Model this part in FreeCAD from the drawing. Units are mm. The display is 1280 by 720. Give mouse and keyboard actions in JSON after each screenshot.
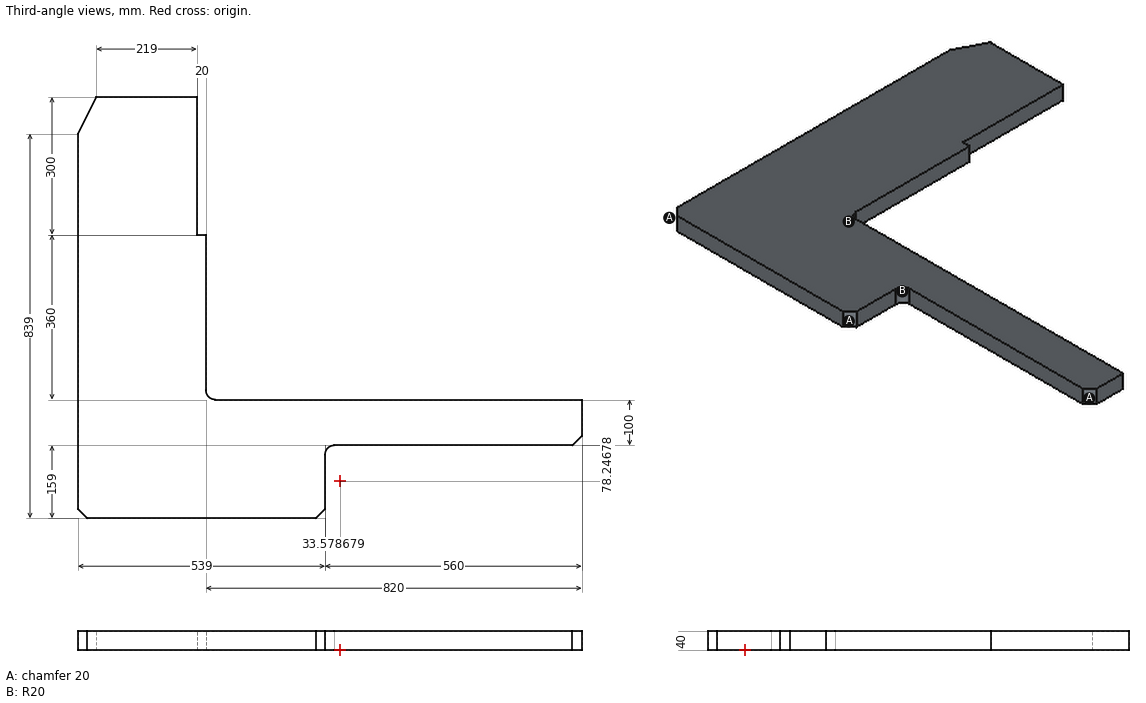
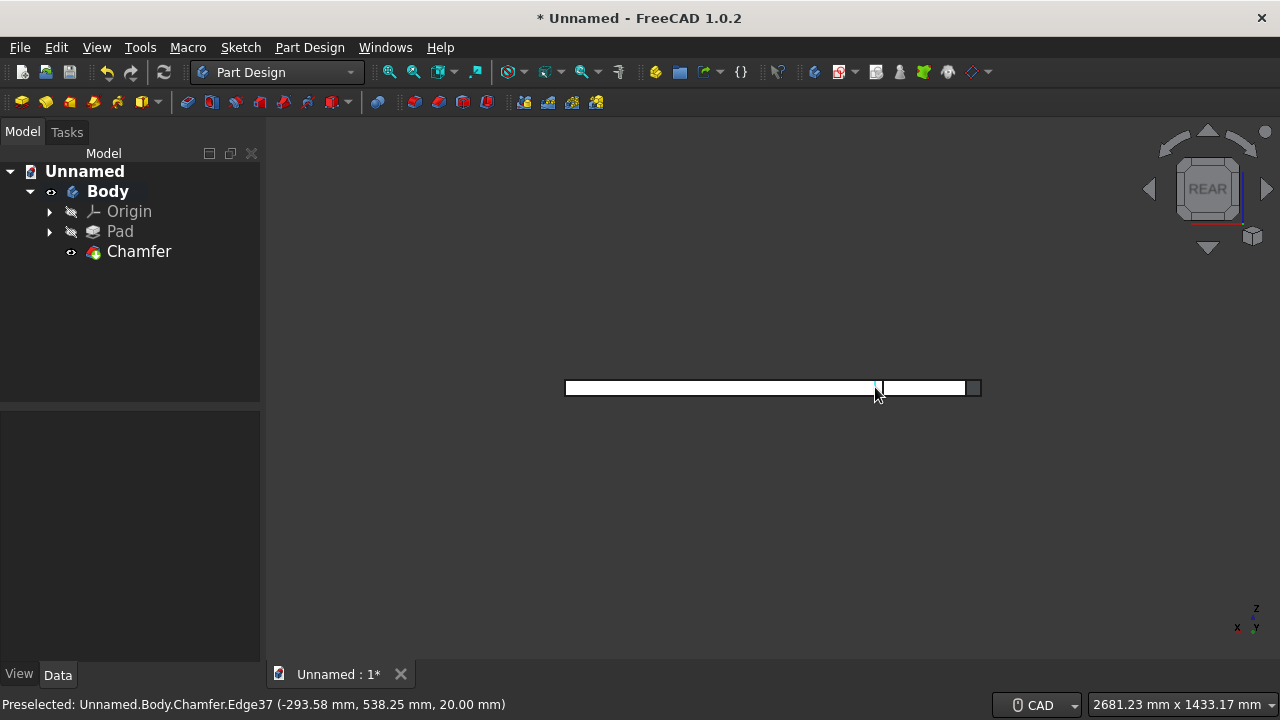
{"action": "key", "text": "6"}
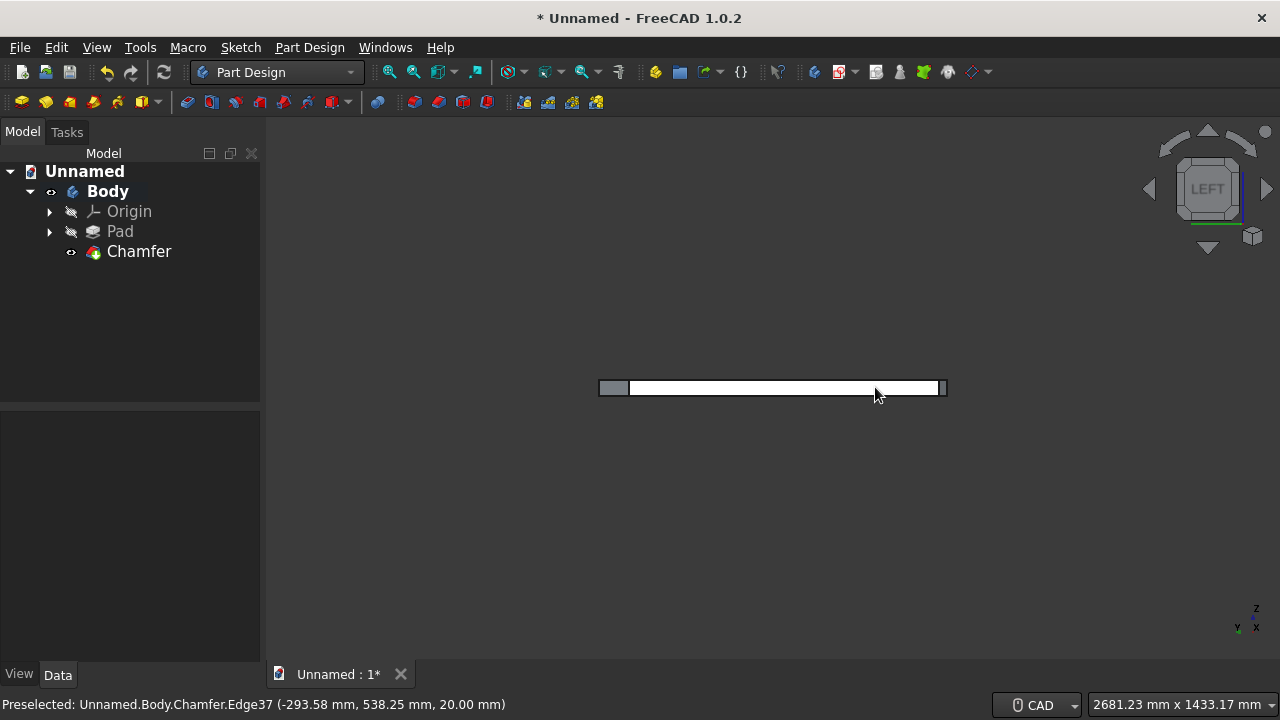
{"action": "key", "text": "v f"}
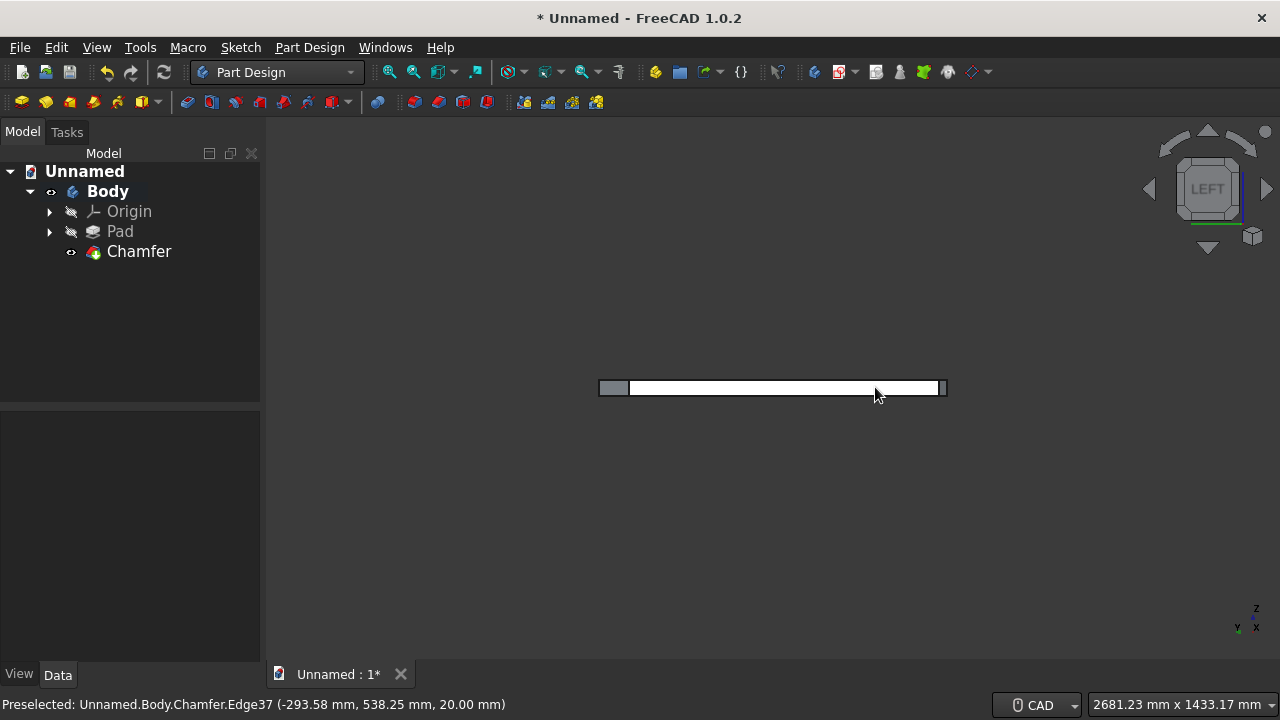
{"action": "scroll", "coordinate": [849, 387], "scroll_direction": "up", "scroll_amount": 5}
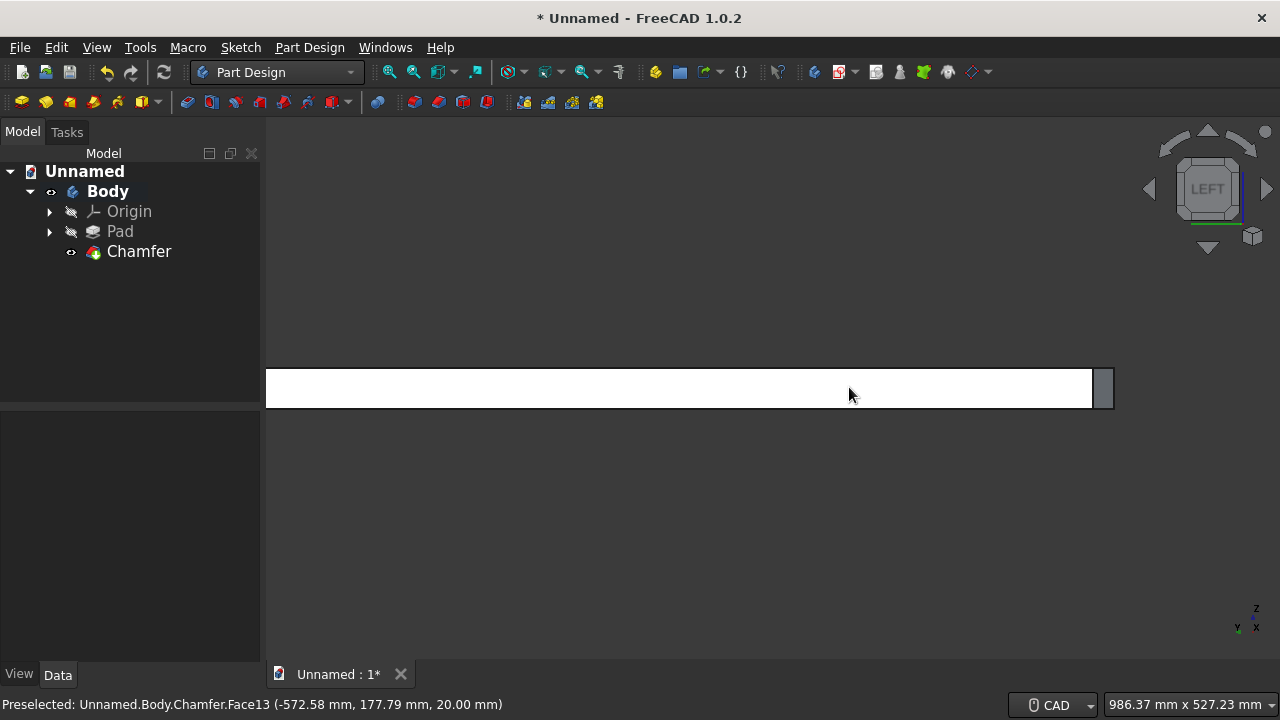
{"action": "key", "text": "v f"}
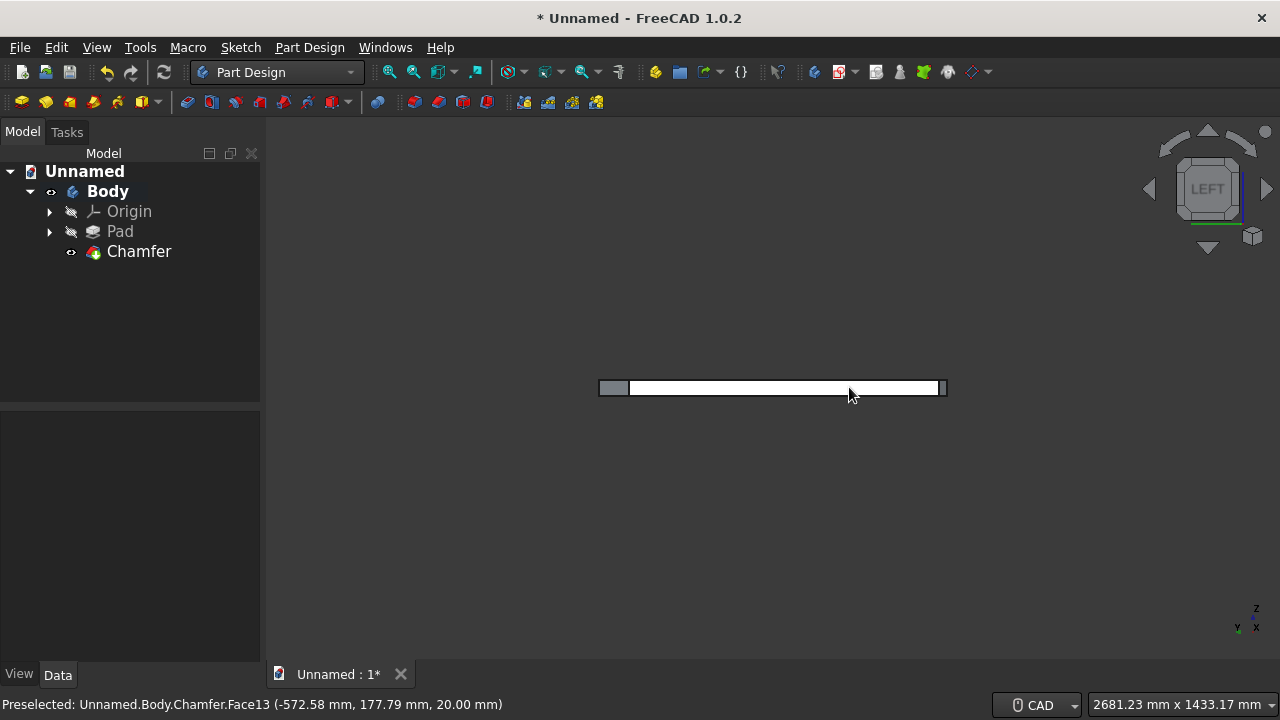
{"action": "key", "text": "v 3"}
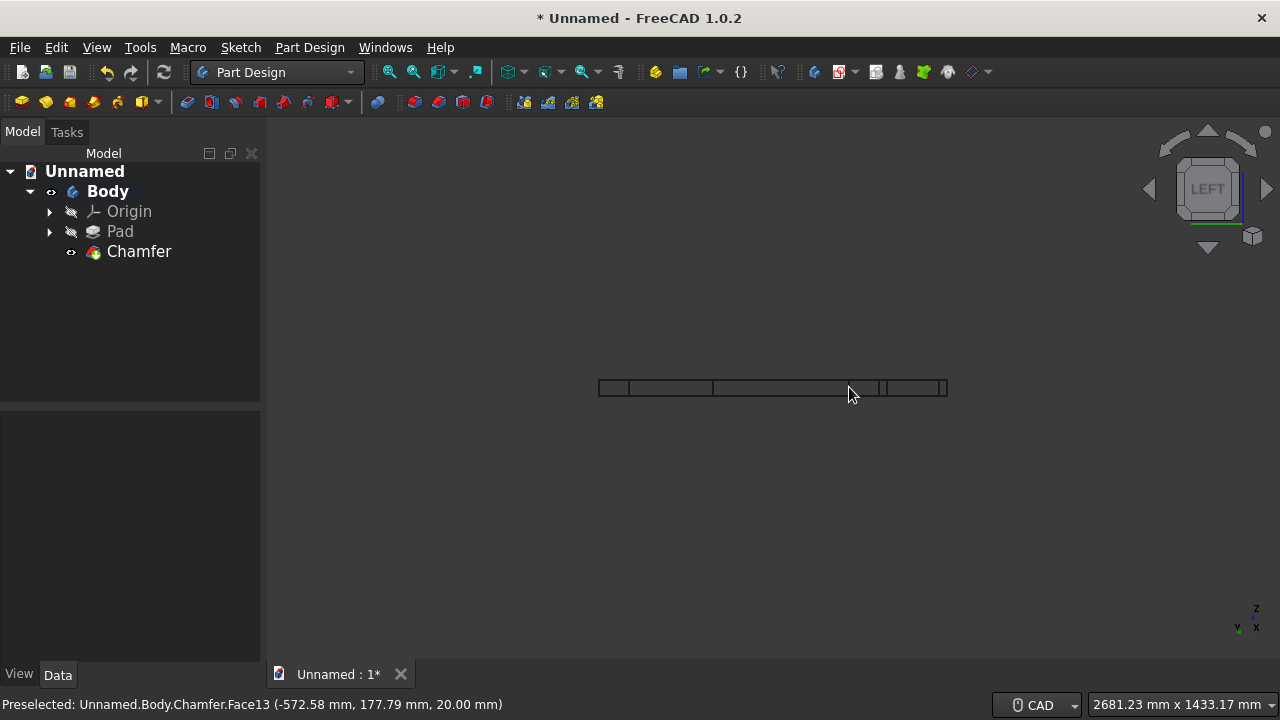
{"action": "key", "text": "0"}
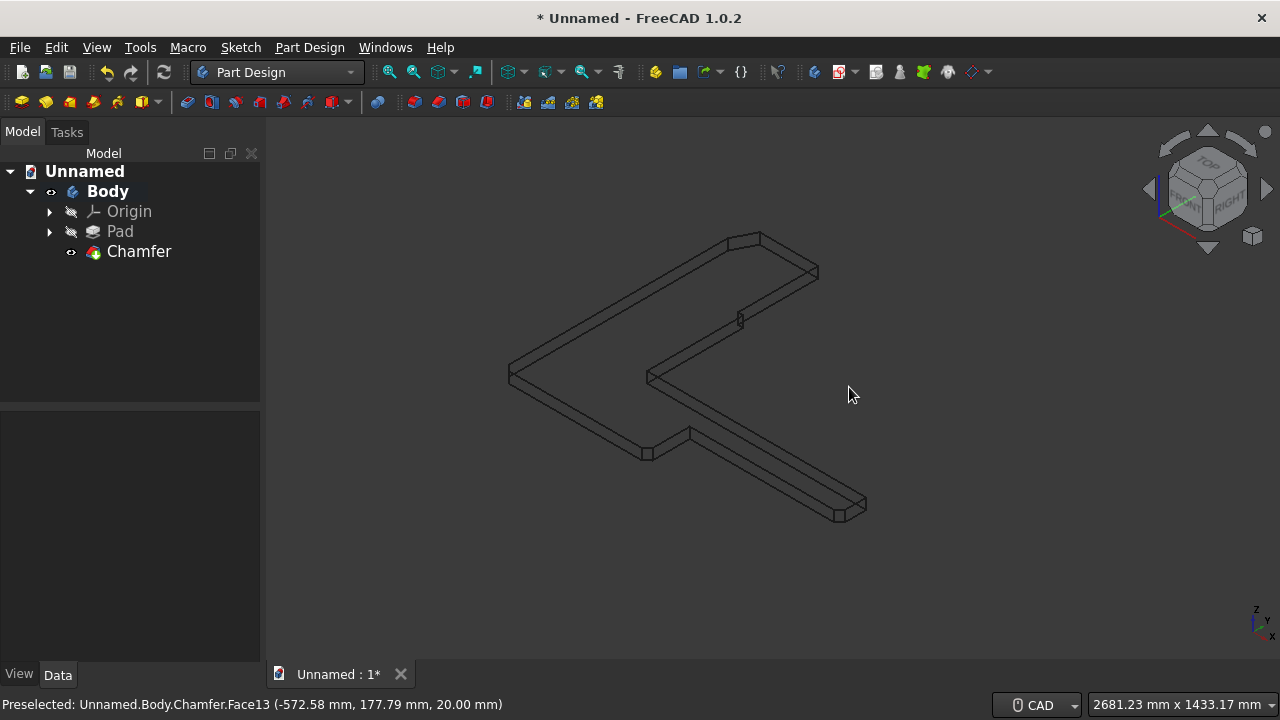
{"action": "left_click", "coordinate": [647, 379]}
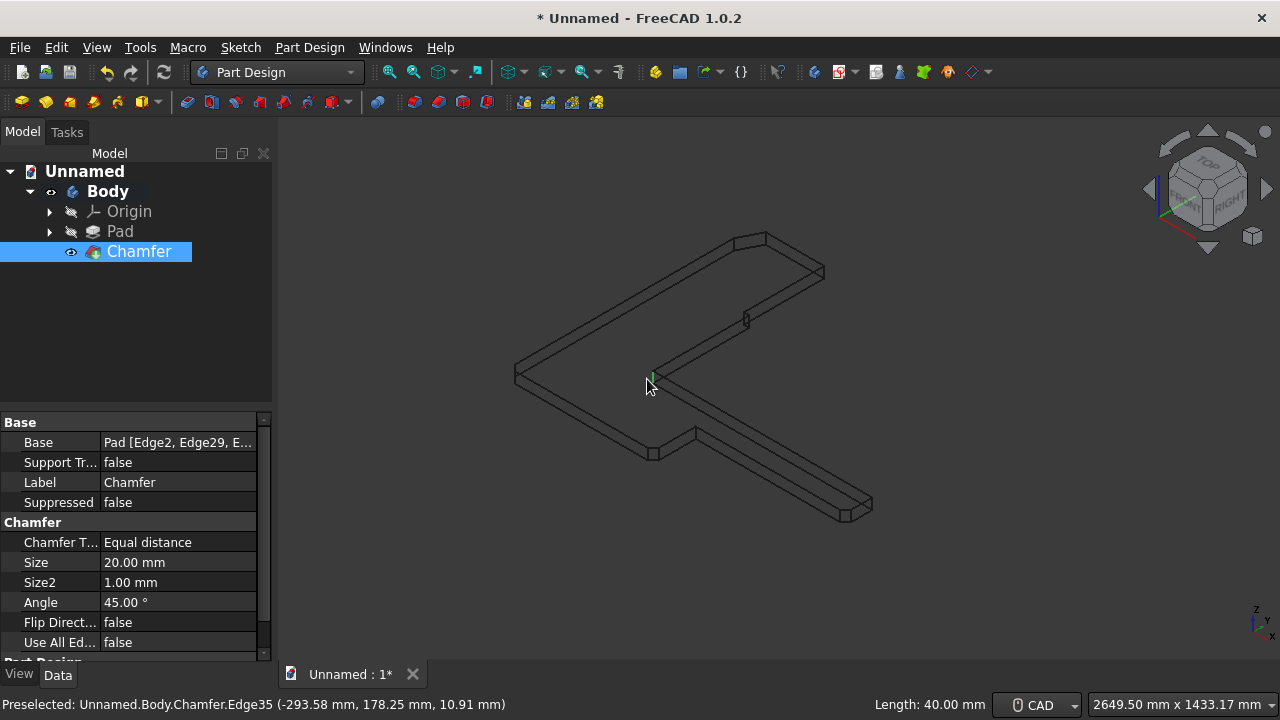
{"action": "left_click", "coordinate": [696, 434], "text": "ctrl"}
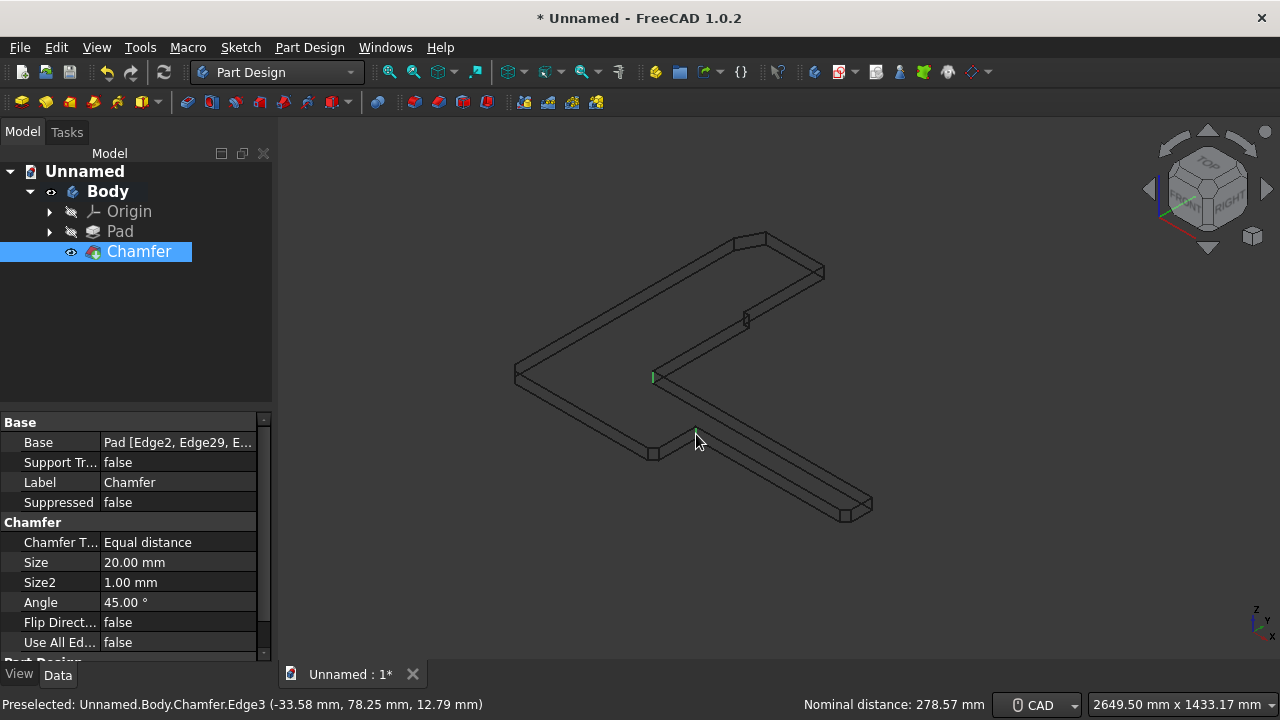
{"action": "key", "text": "v 1"}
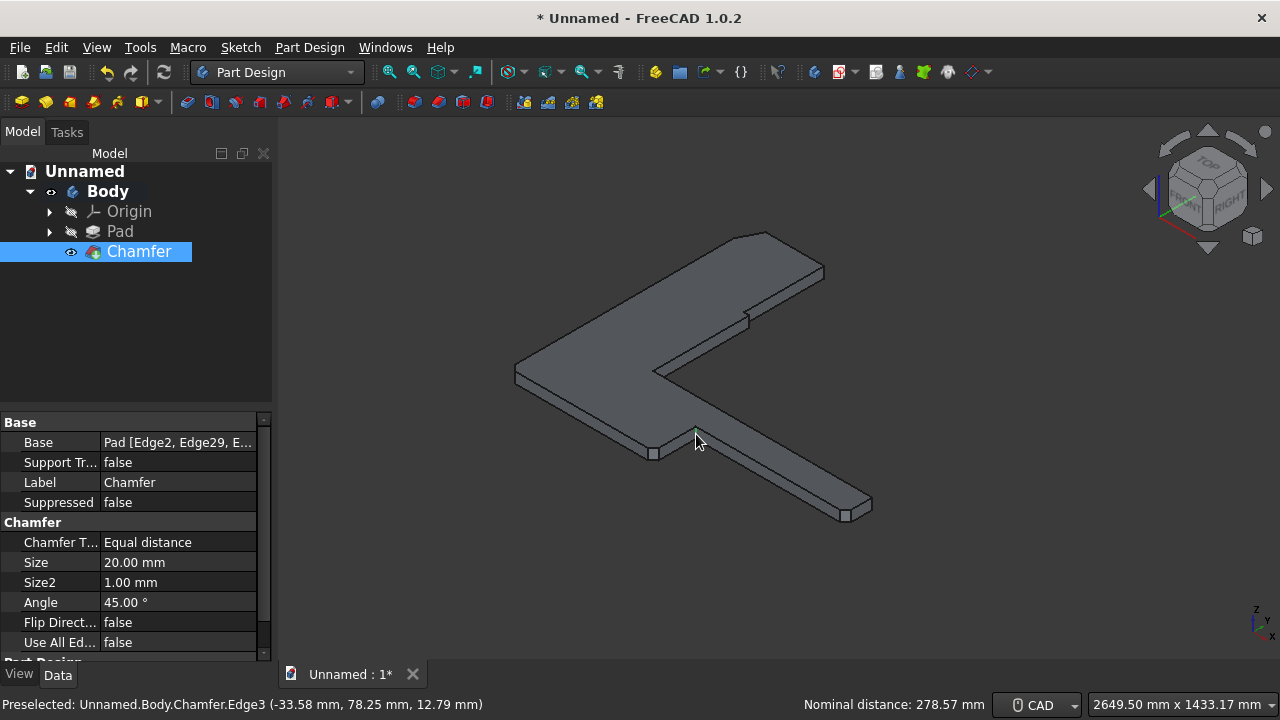
{"action": "left_click", "coordinate": [416, 102]}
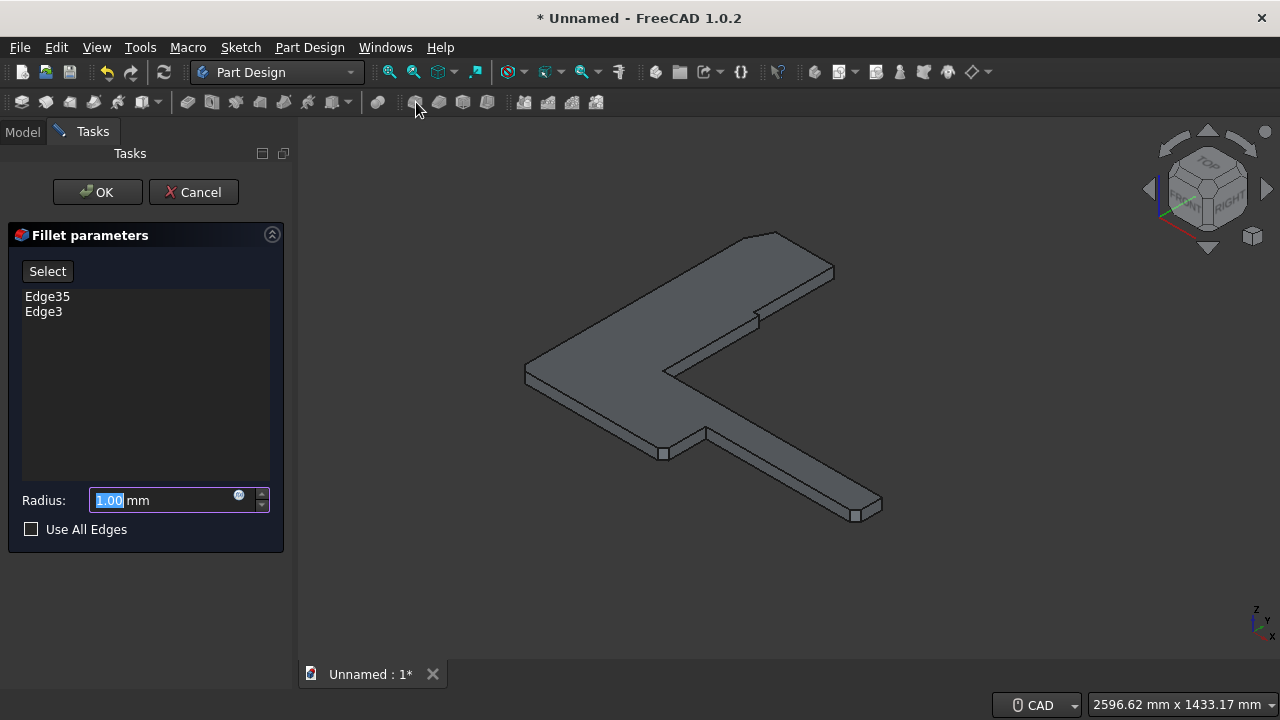
{"action": "type", "text": "20"}
{"action": "key", "text": "Tab"}